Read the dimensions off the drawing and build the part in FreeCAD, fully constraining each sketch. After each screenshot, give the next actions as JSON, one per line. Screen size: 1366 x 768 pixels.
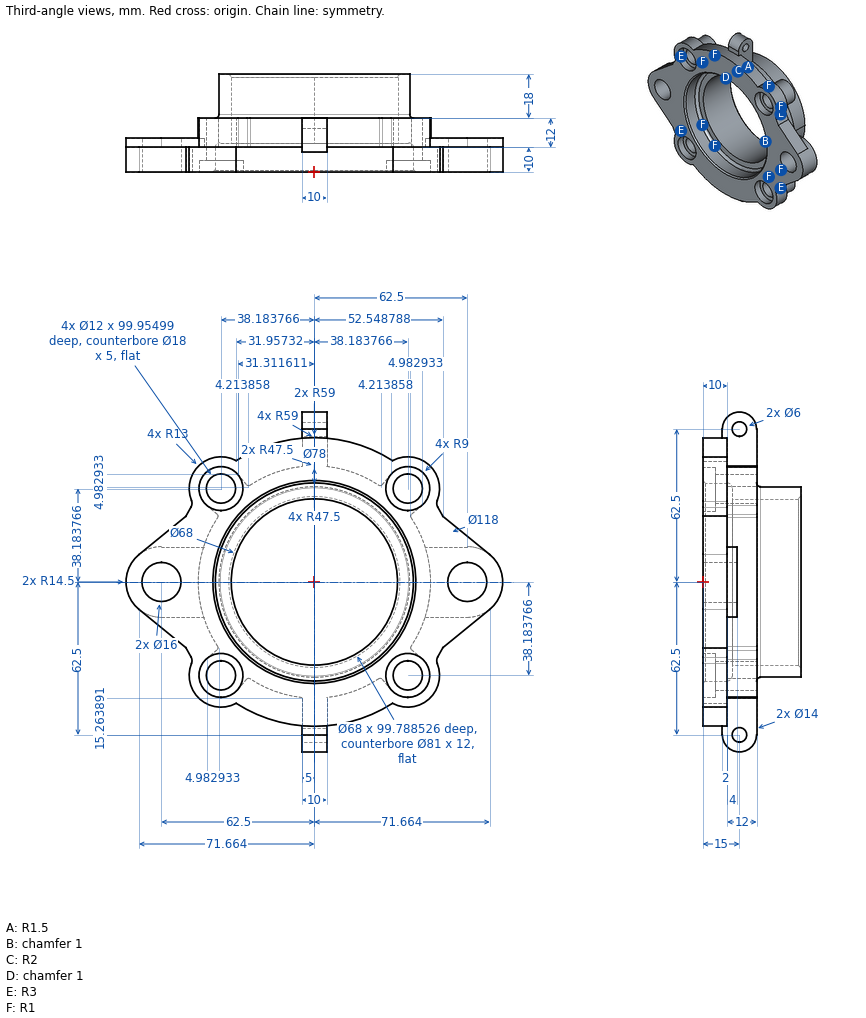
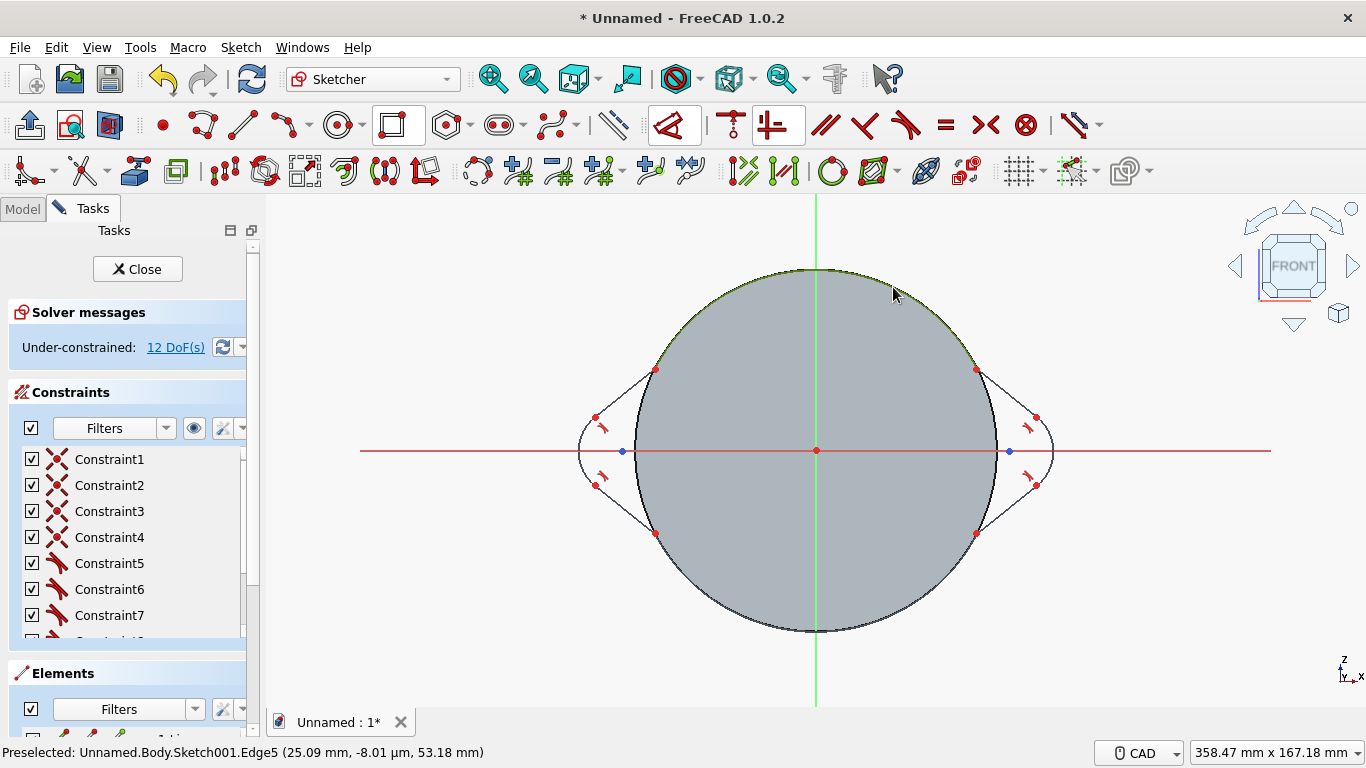
{"action": "left_click", "coordinate": [739, 615]}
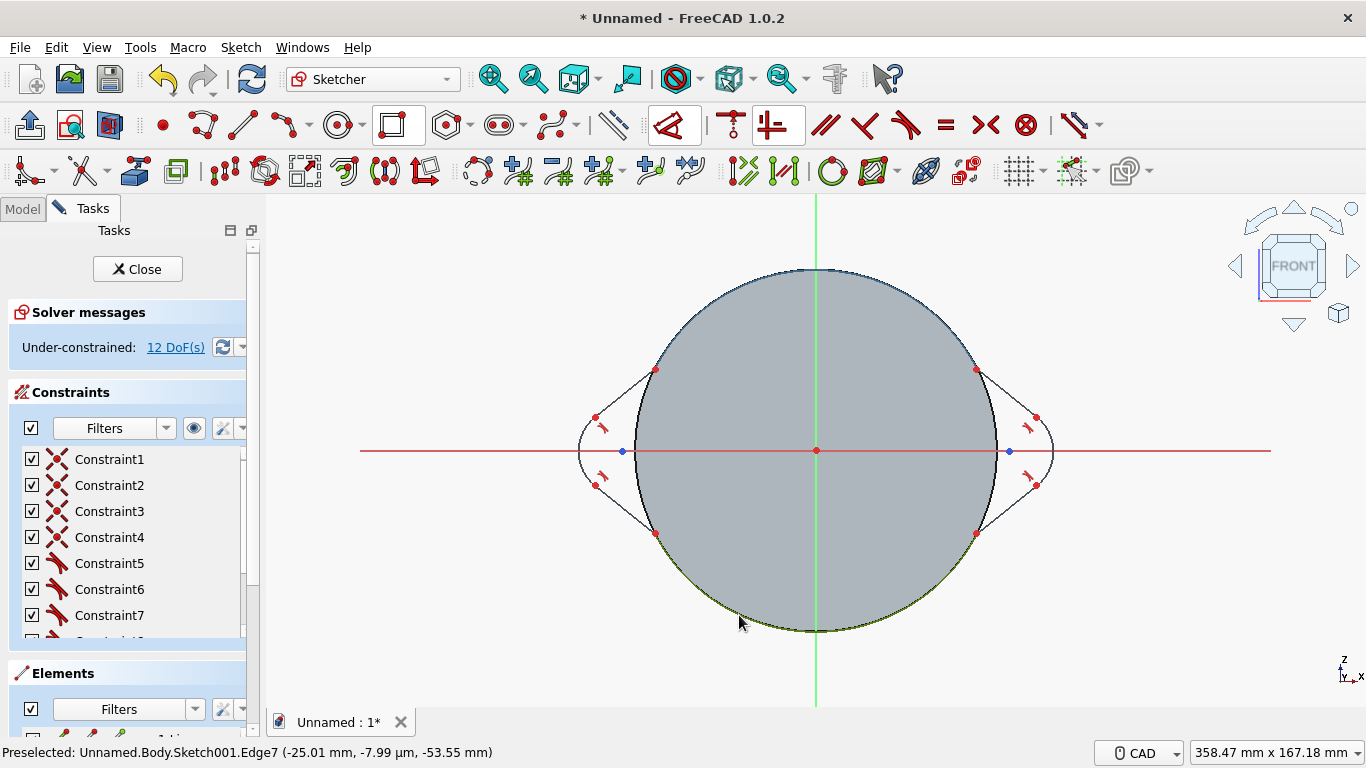
{"action": "left_click", "coordinate": [946, 126]}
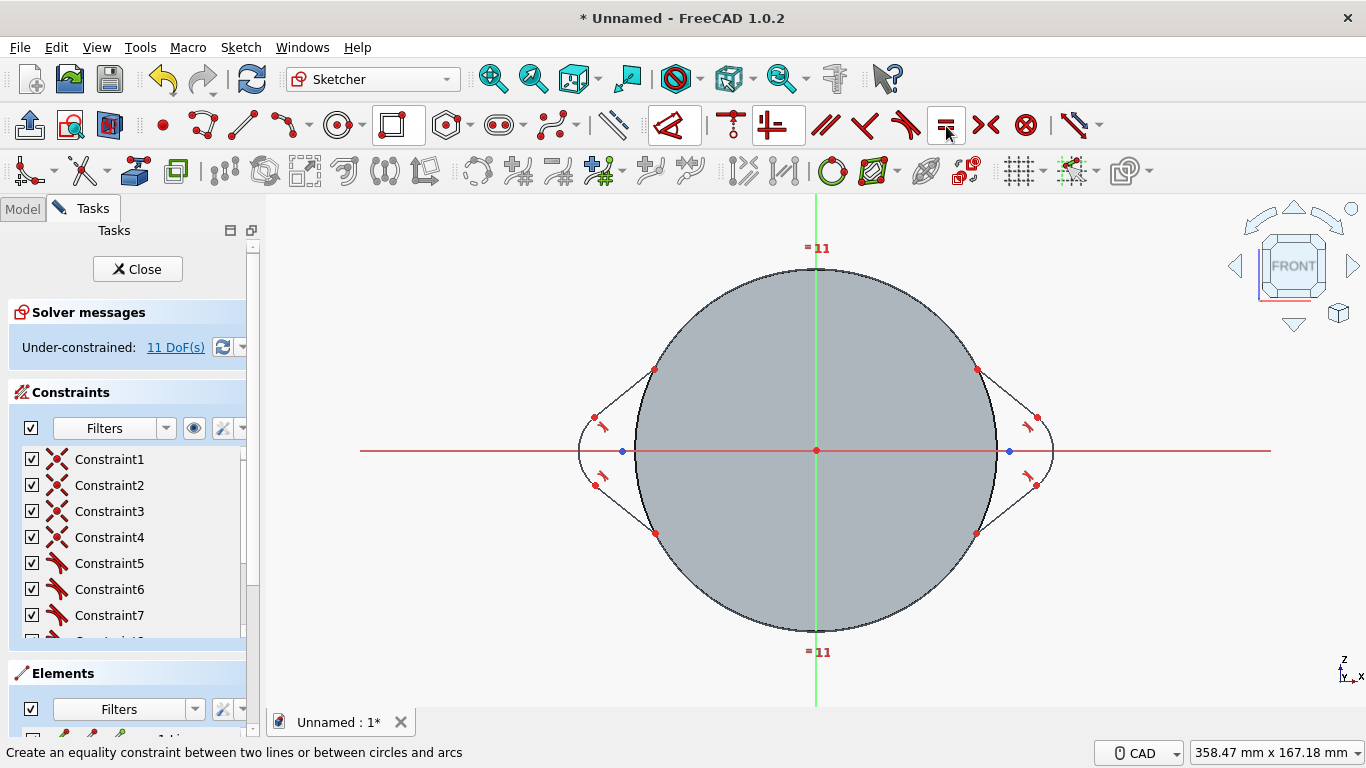
{"action": "left_click", "coordinate": [581, 436]}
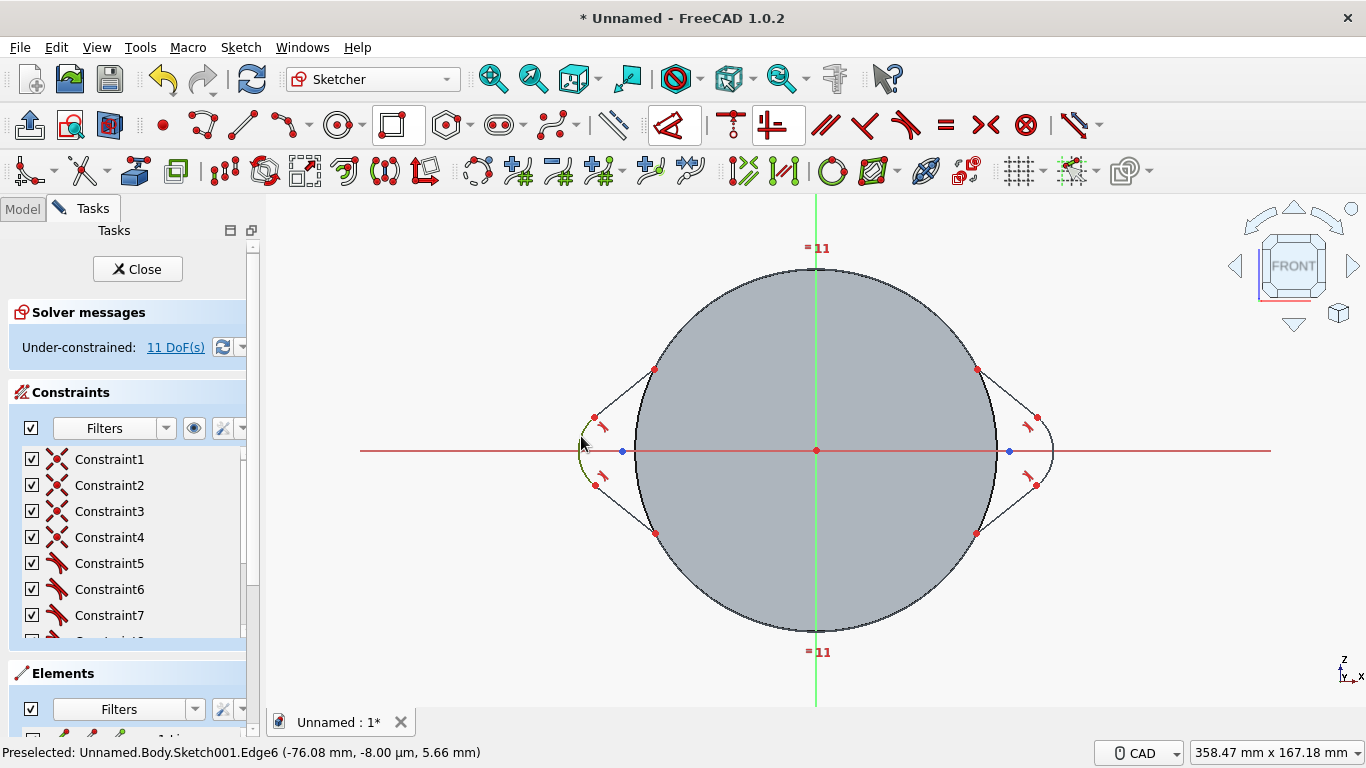
{"action": "left_click", "coordinate": [1051, 467]}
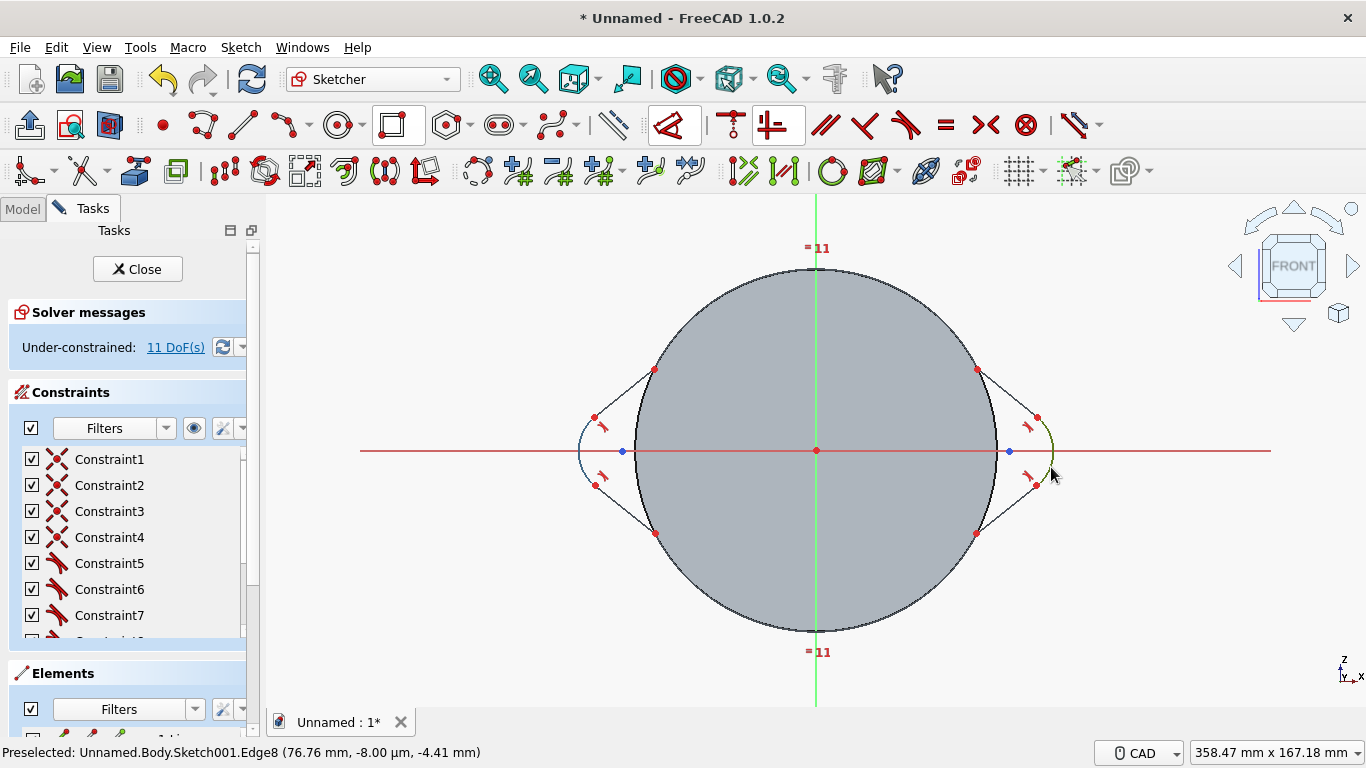
{"action": "left_click", "coordinate": [946, 126]}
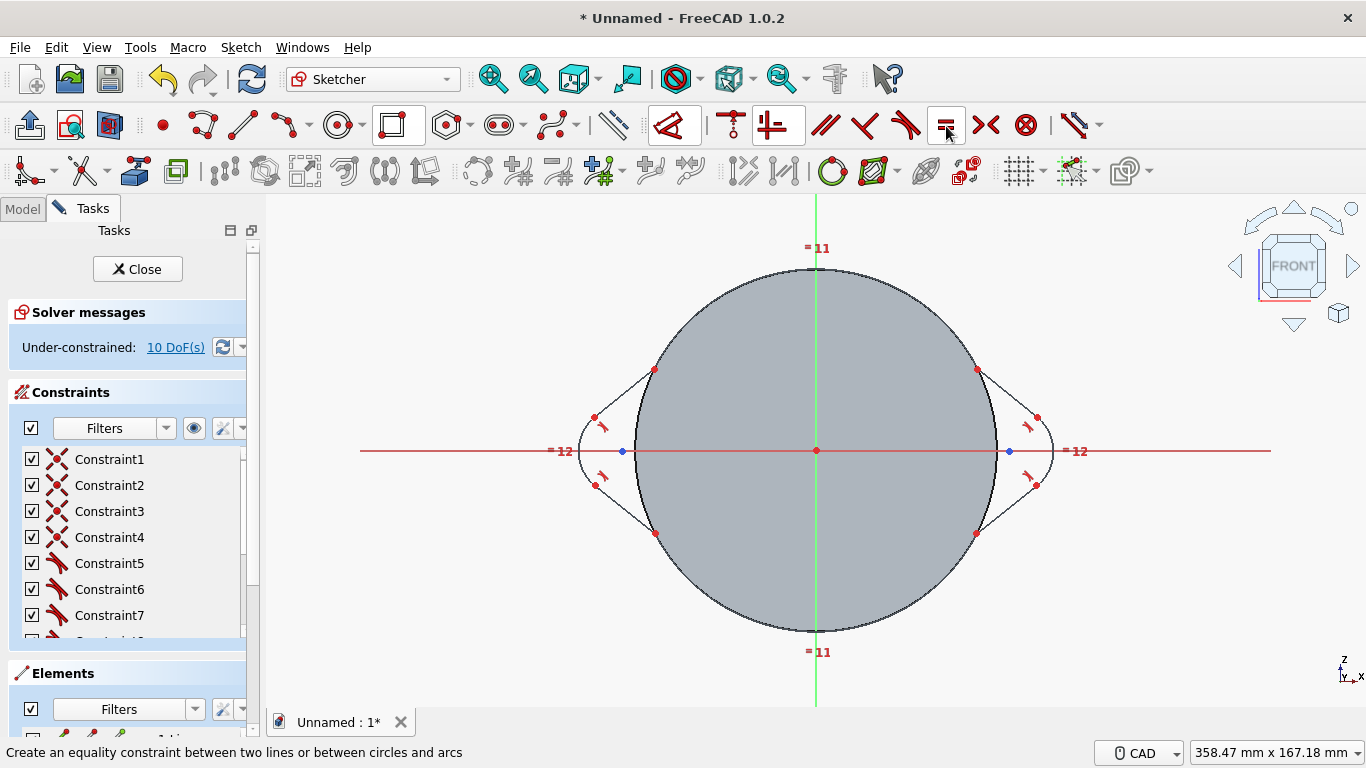
{"action": "left_click", "coordinate": [623, 451]}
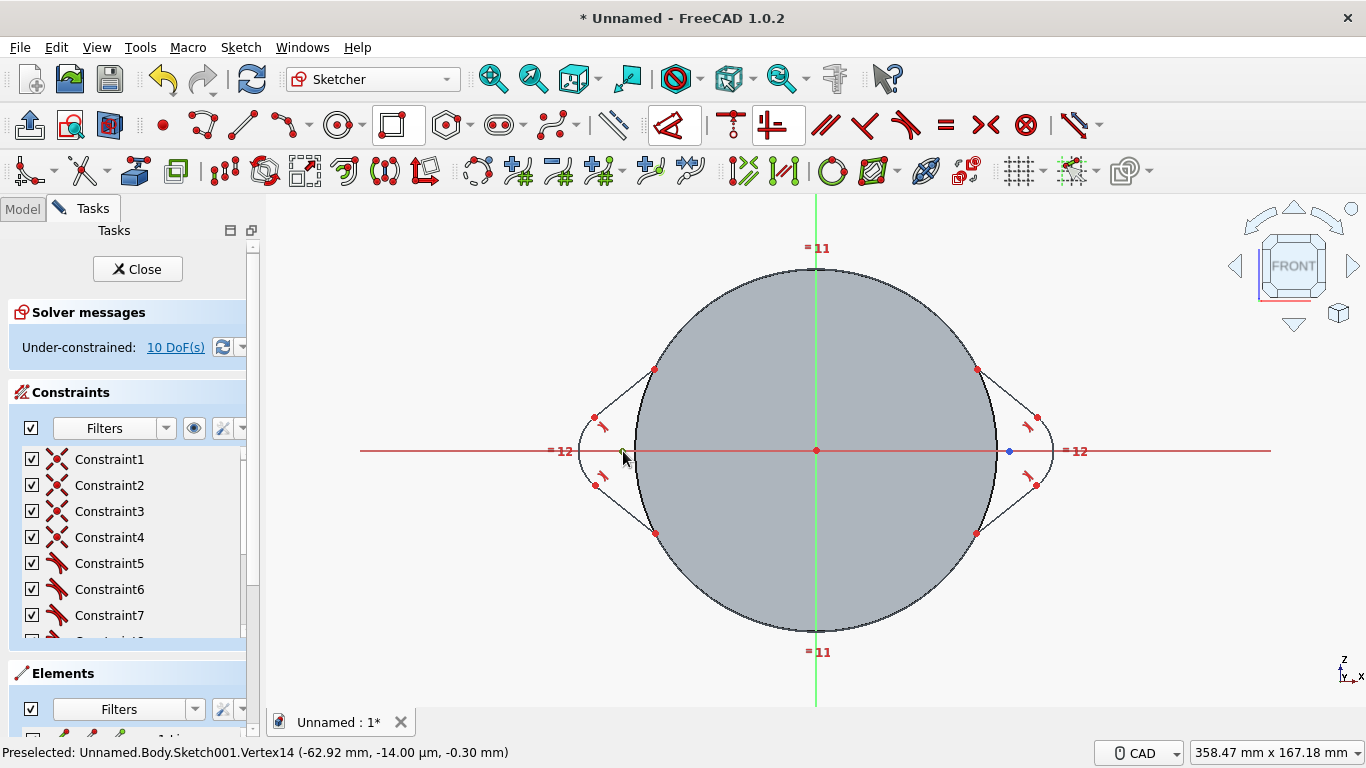
{"action": "left_click", "coordinate": [359, 450]}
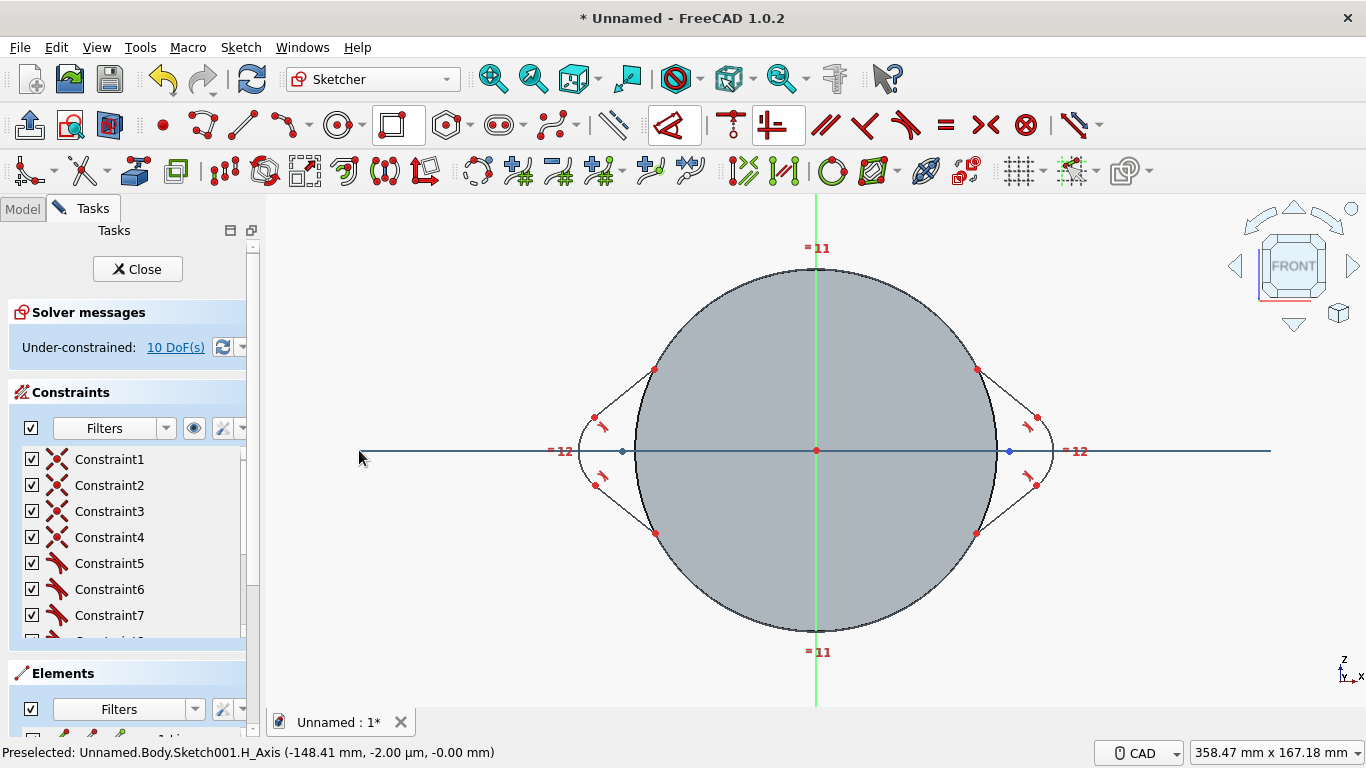
{"action": "left_click", "coordinate": [732, 126]}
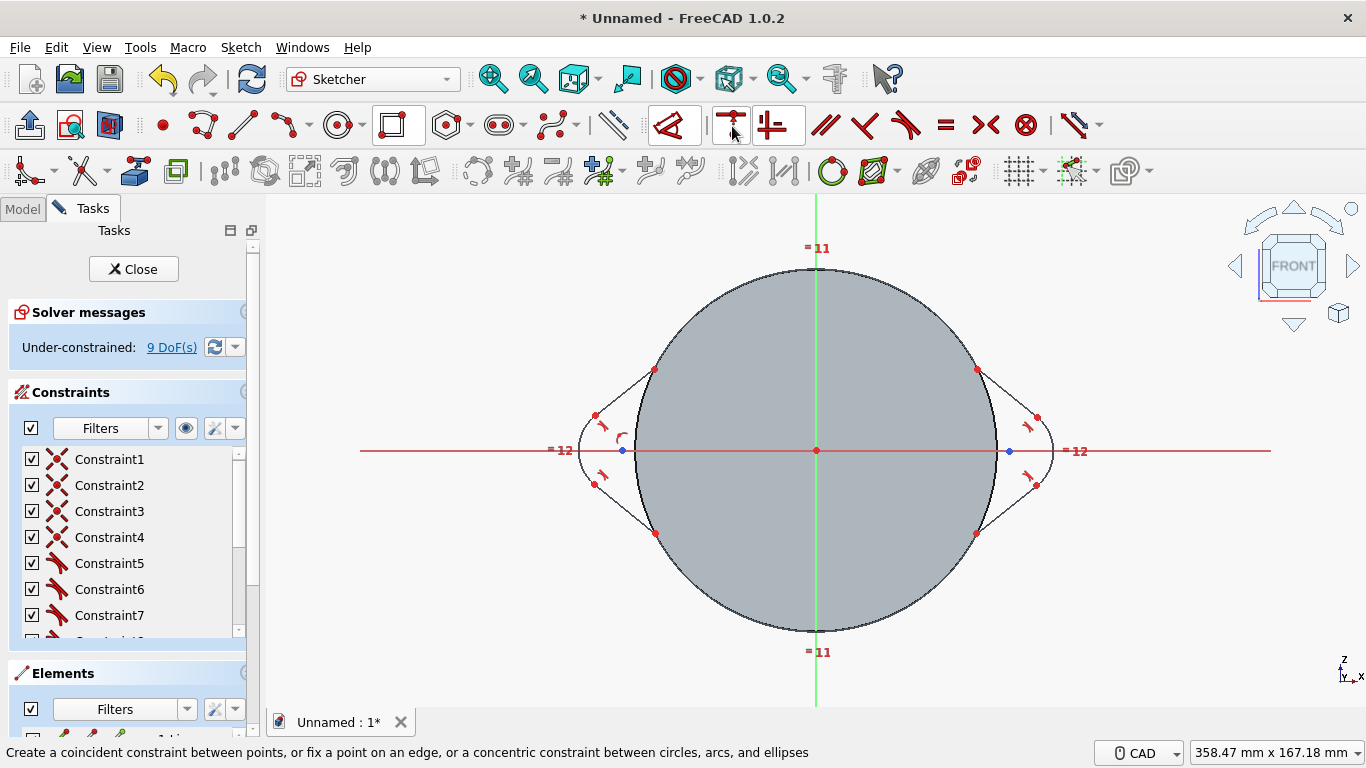
{"action": "left_click", "coordinate": [1009, 451]}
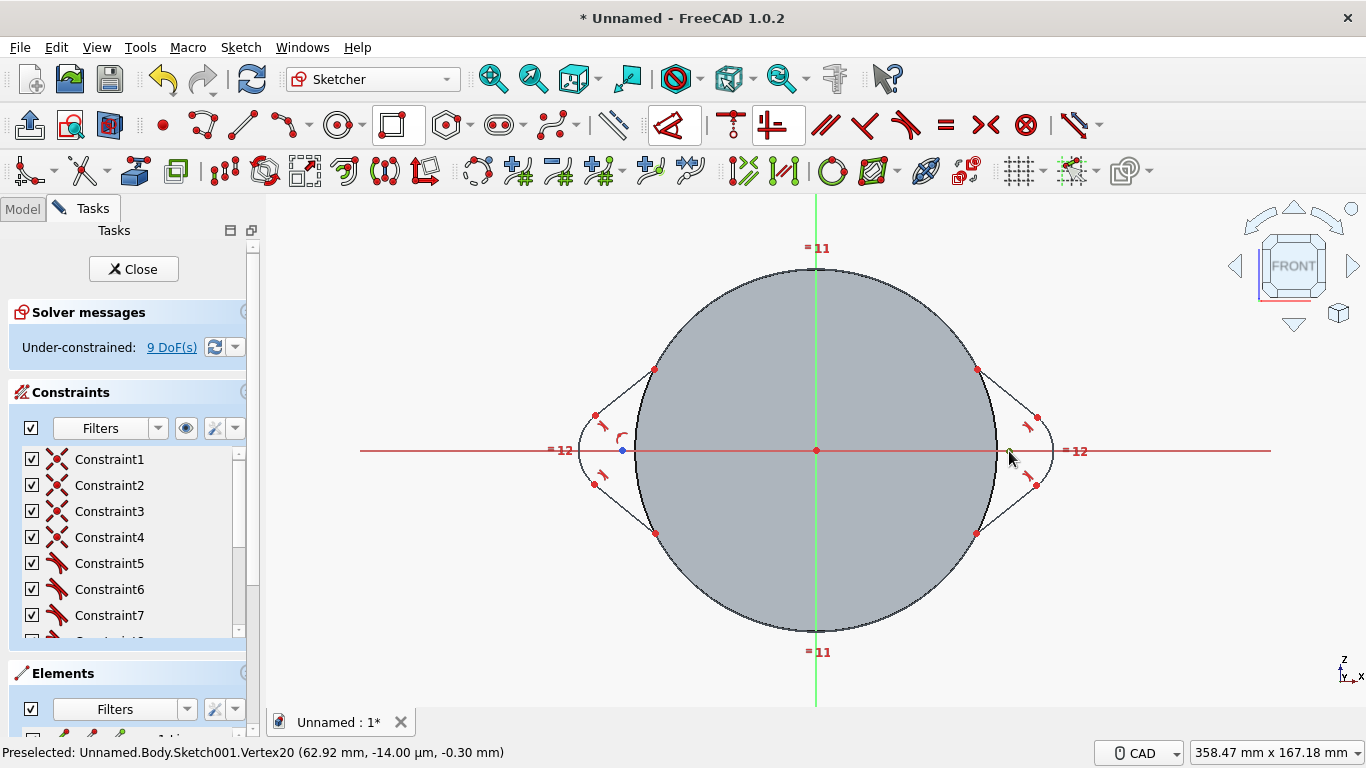
{"action": "left_click", "coordinate": [359, 450]}